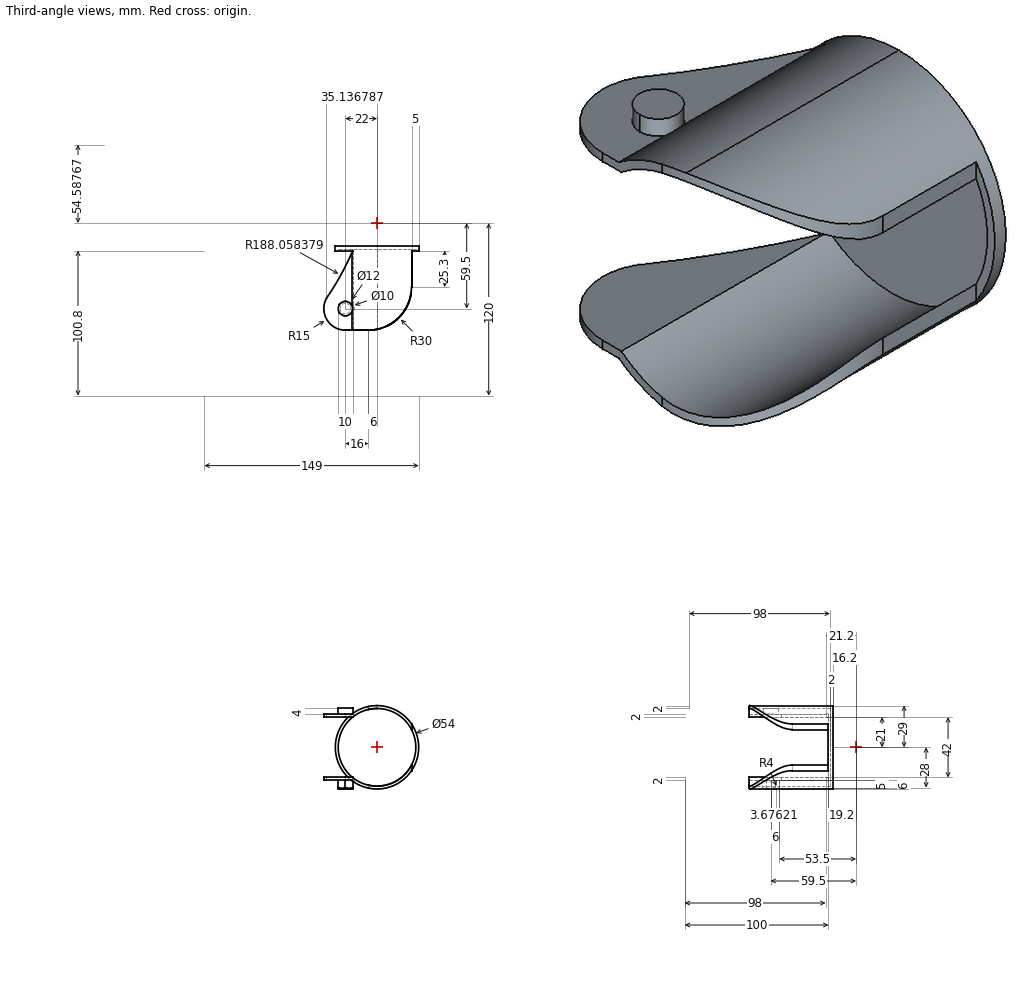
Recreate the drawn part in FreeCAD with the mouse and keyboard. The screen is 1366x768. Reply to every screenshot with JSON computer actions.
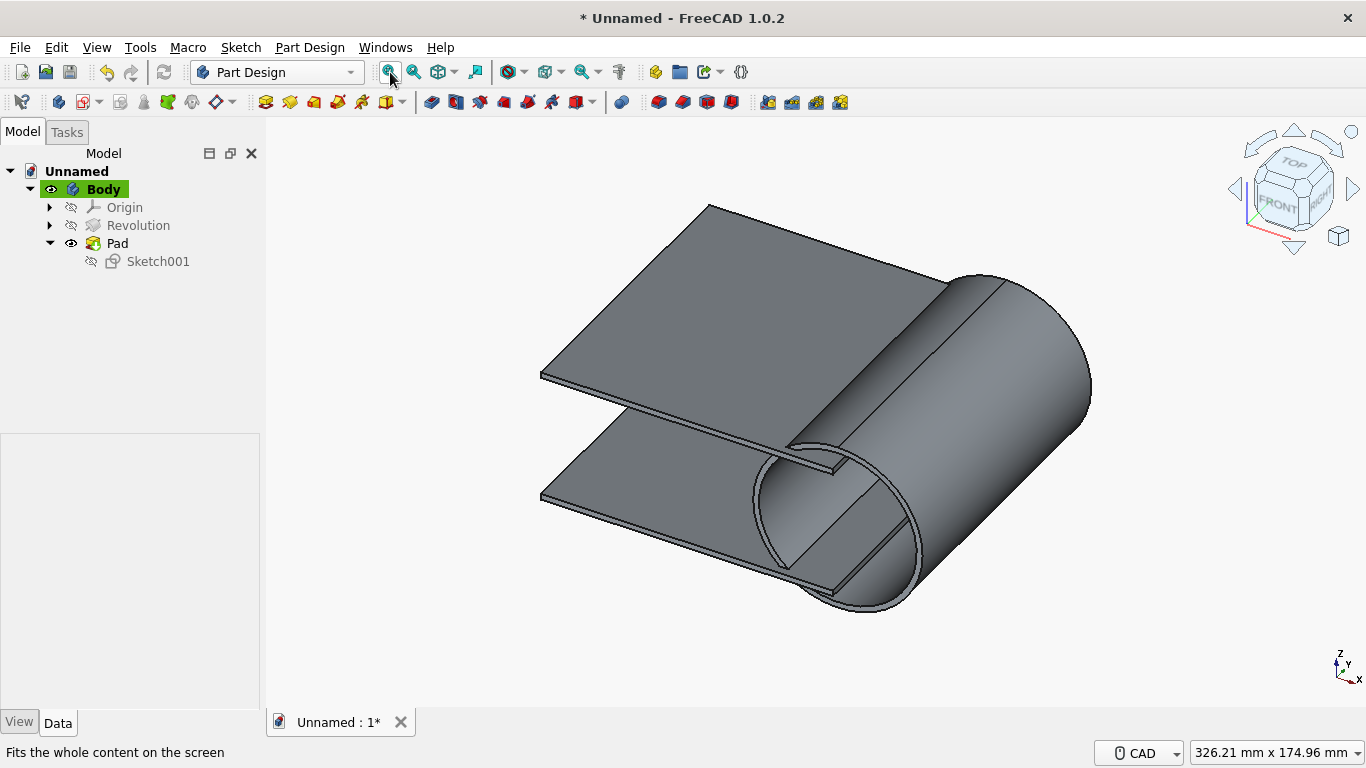
{"action": "left_click", "coordinate": [84, 102]}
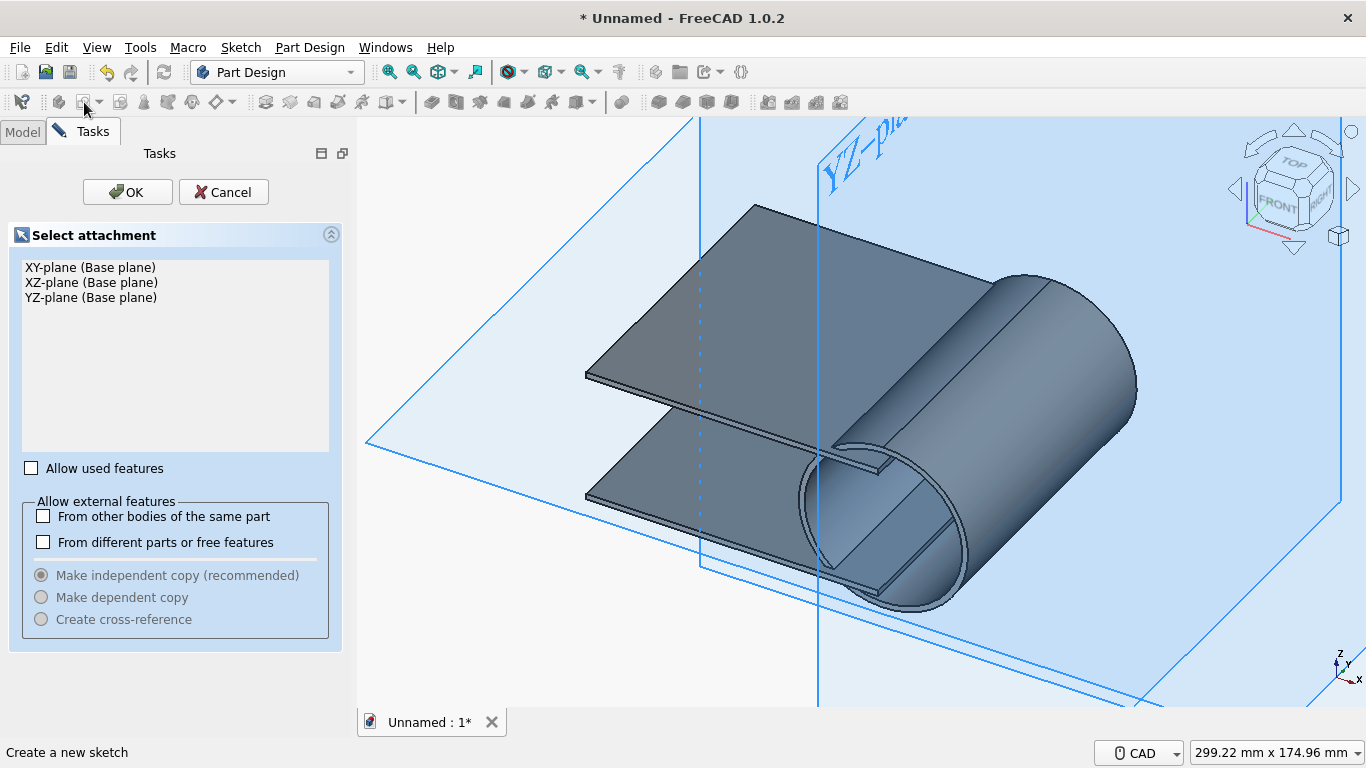
{"action": "left_click", "coordinate": [82, 298]}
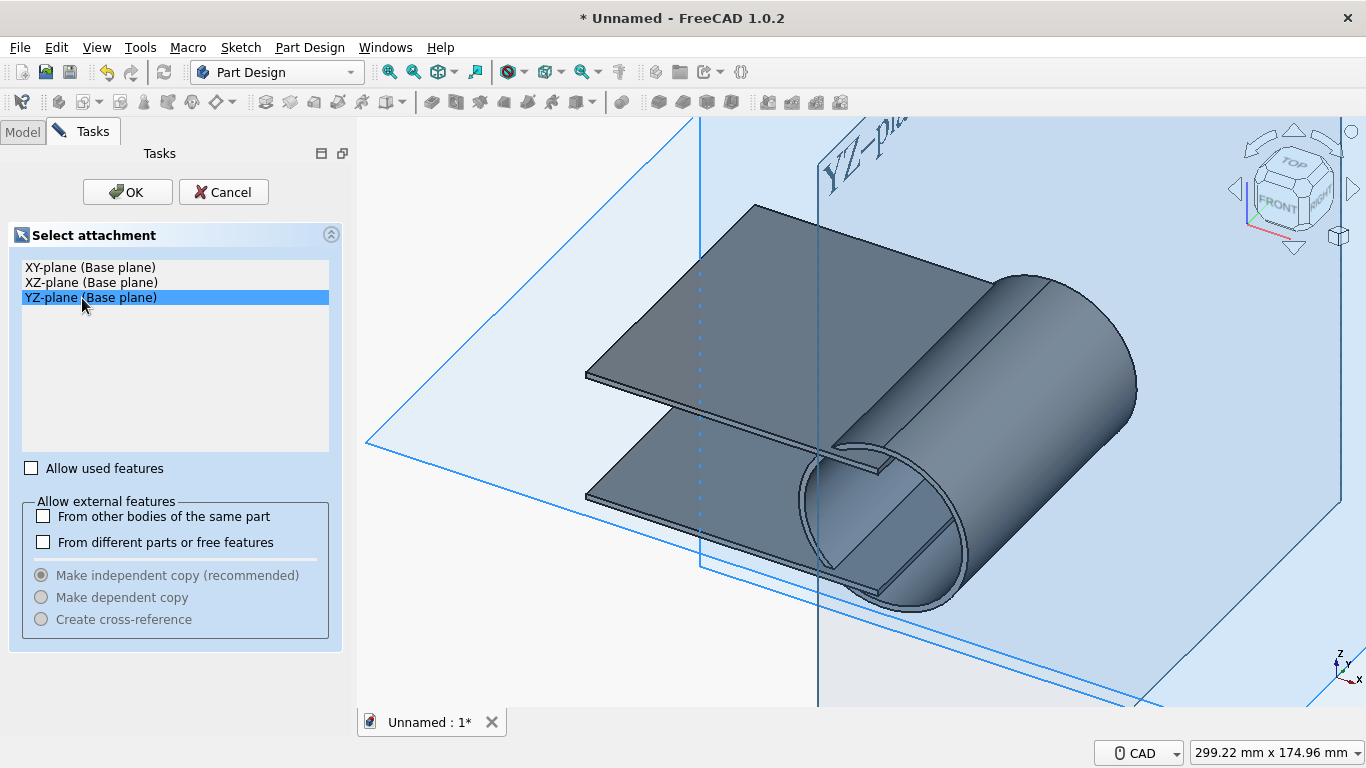
{"action": "left_click", "coordinate": [128, 192]}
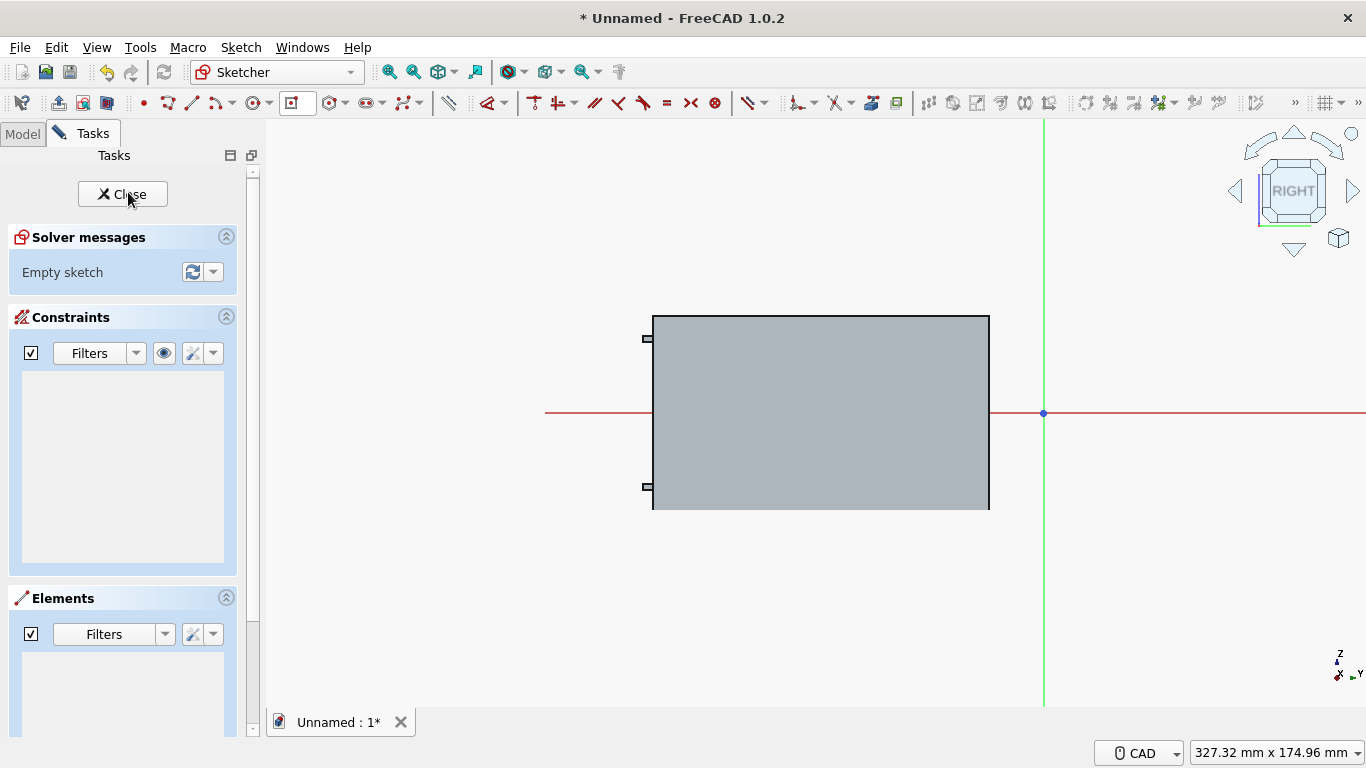
{"action": "left_click", "coordinate": [108, 104]}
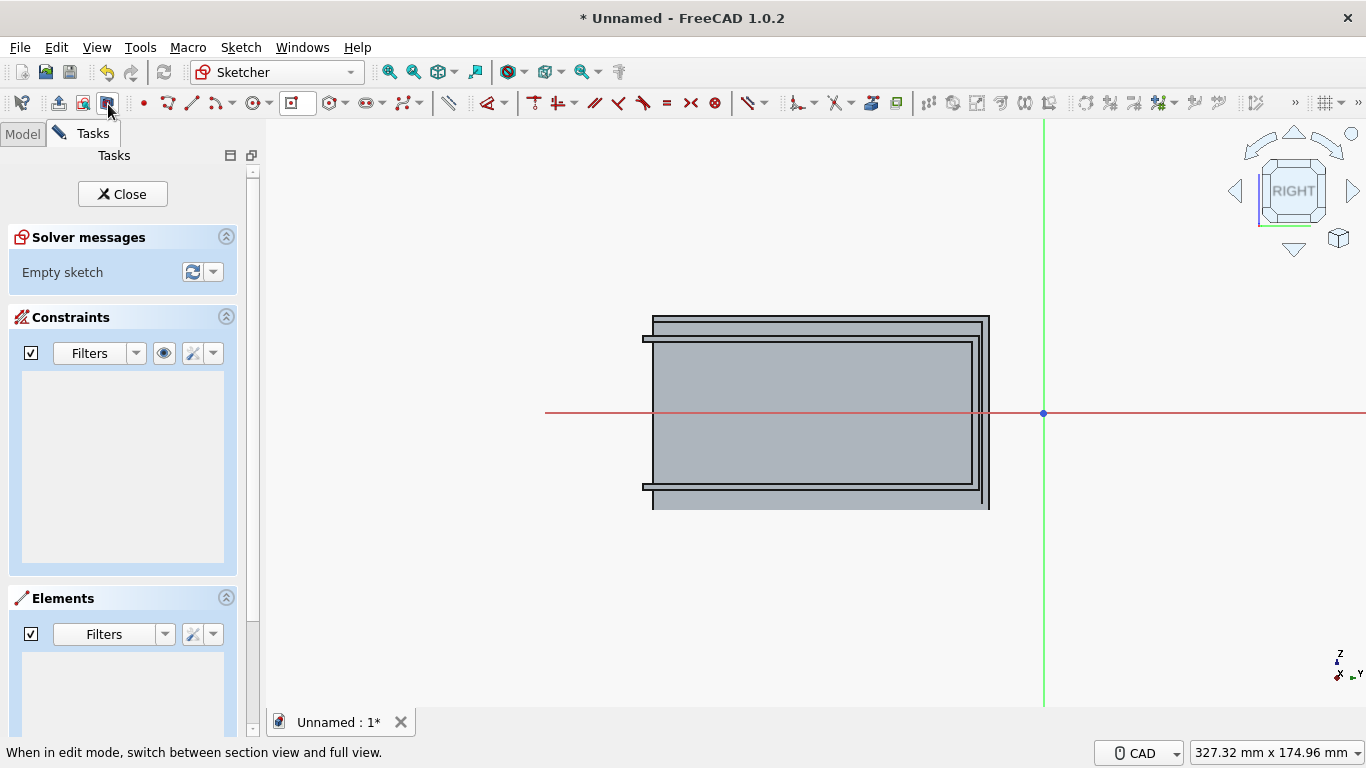
{"action": "scroll", "coordinate": [1038, 413], "scroll_direction": "up", "scroll_amount": 2}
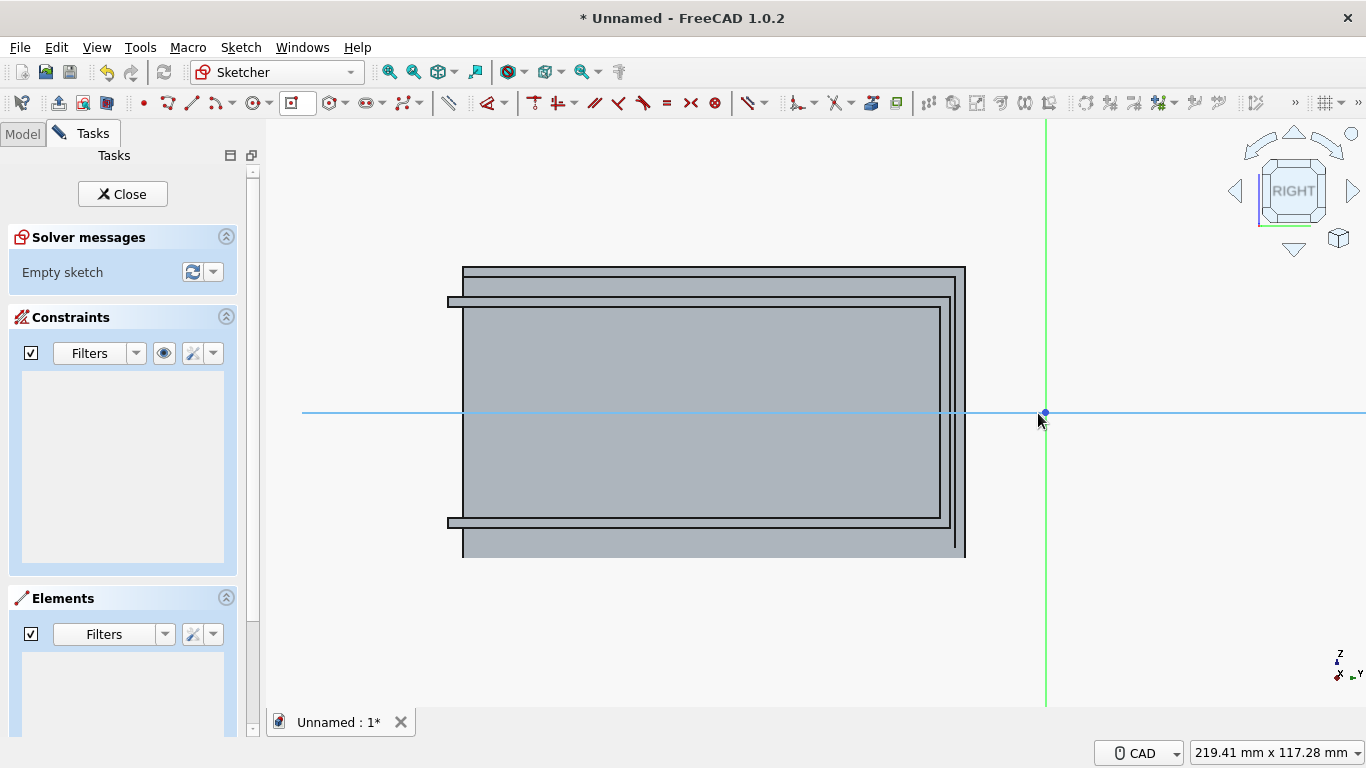
{"action": "key", "text": "g r"}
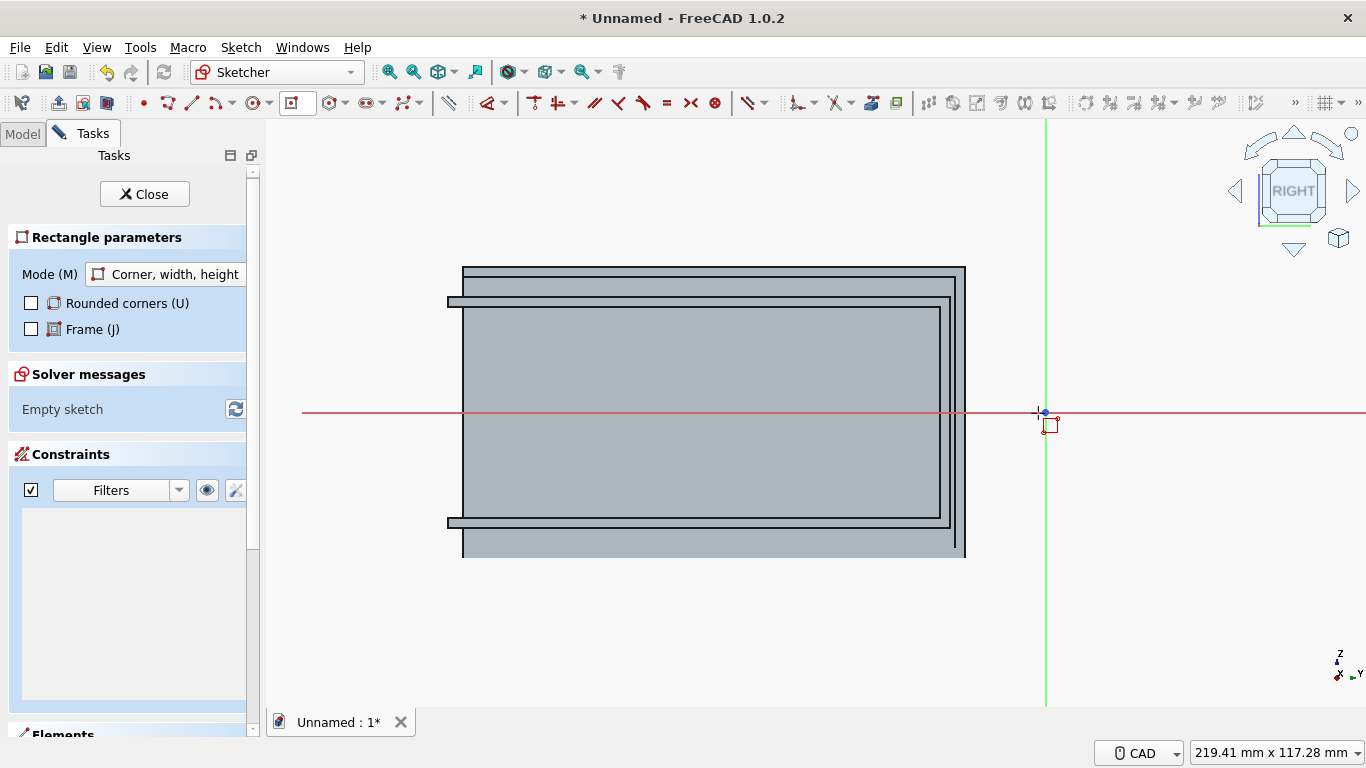
{"action": "left_click", "coordinate": [448, 307]}
{"action": "left_click", "coordinate": [950, 518]}
{"action": "key", "text": "Escape"}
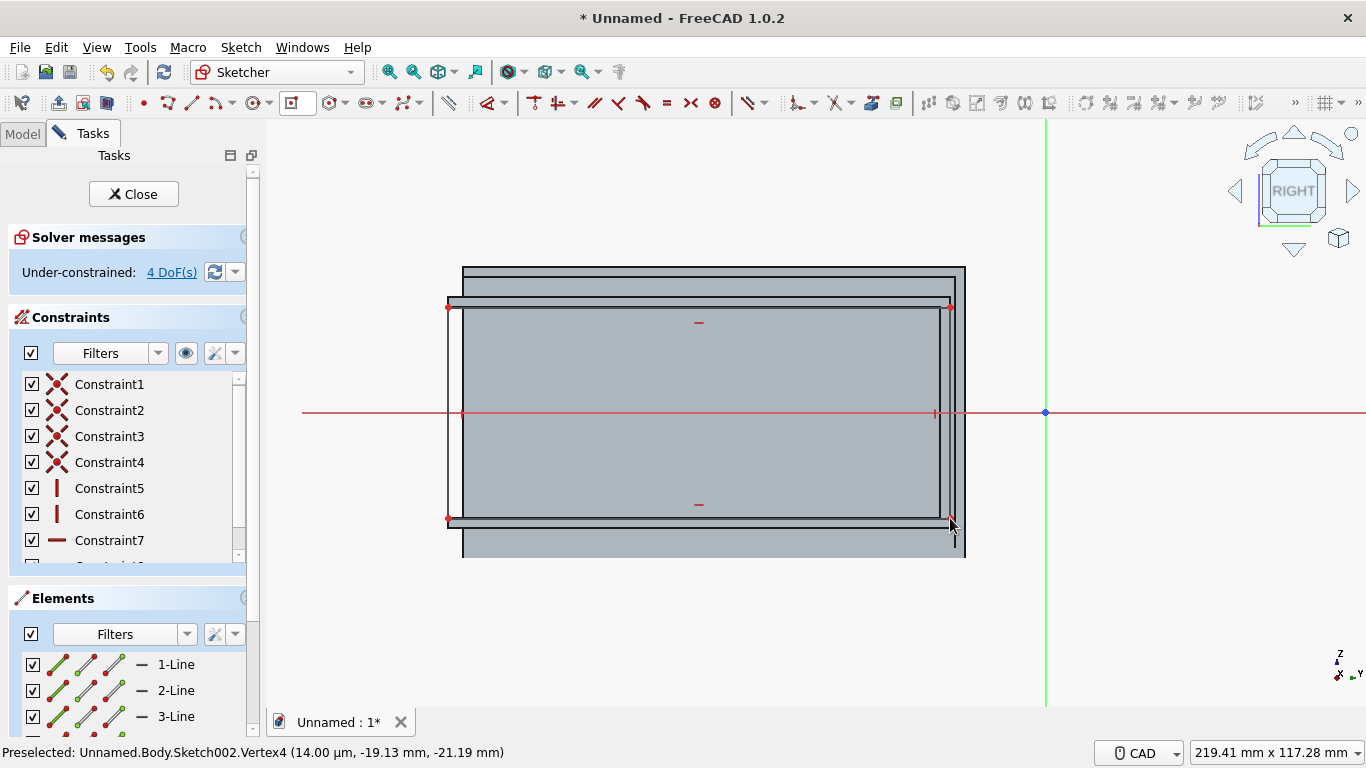
{"action": "left_click", "coordinate": [488, 104]}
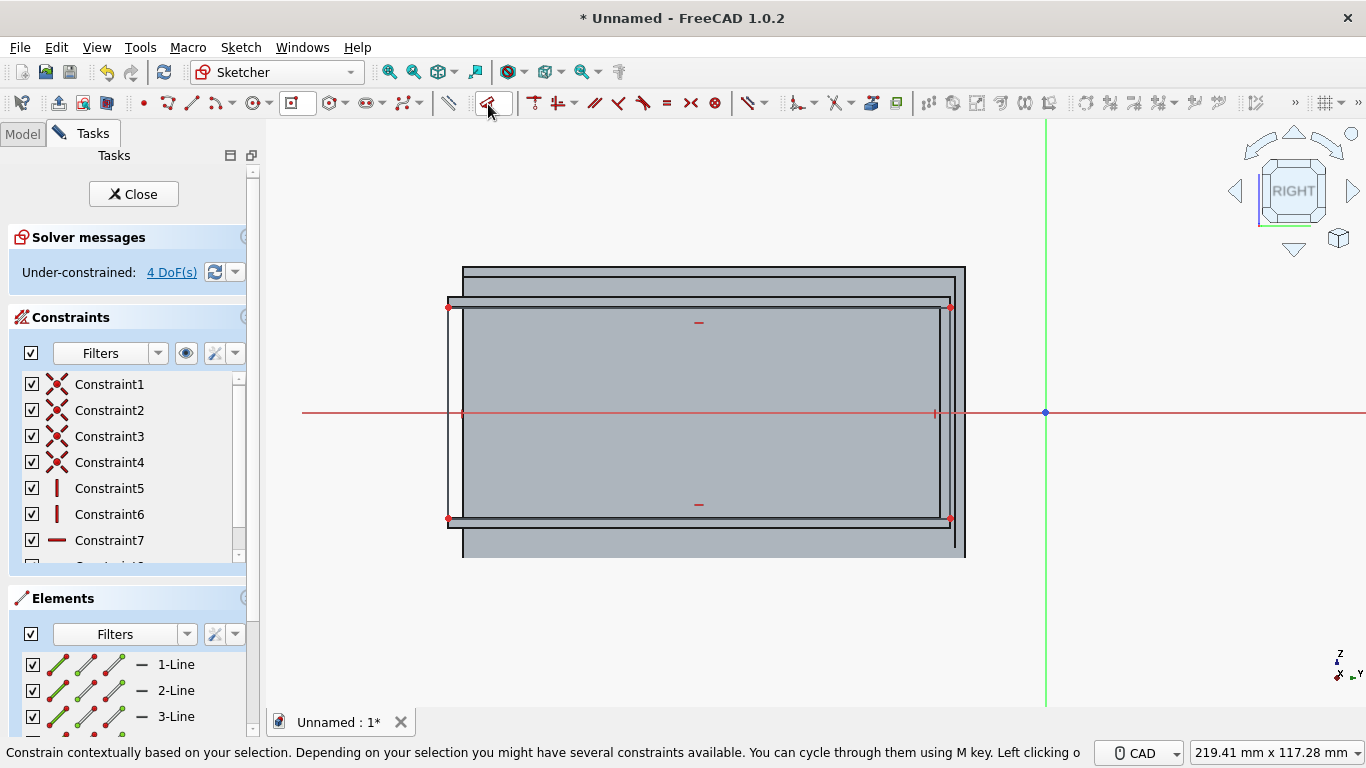
{"action": "left_click", "coordinate": [448, 371]}
{"action": "left_click", "coordinate": [414, 365]}